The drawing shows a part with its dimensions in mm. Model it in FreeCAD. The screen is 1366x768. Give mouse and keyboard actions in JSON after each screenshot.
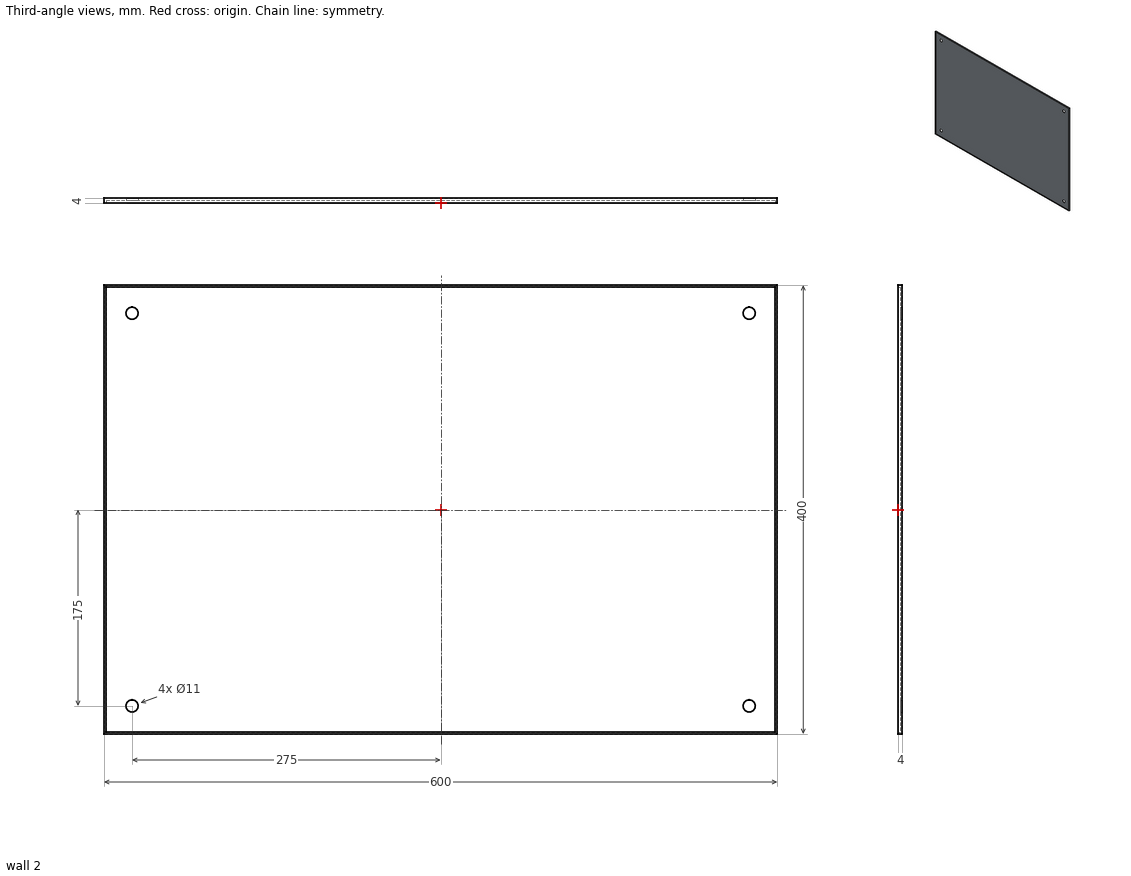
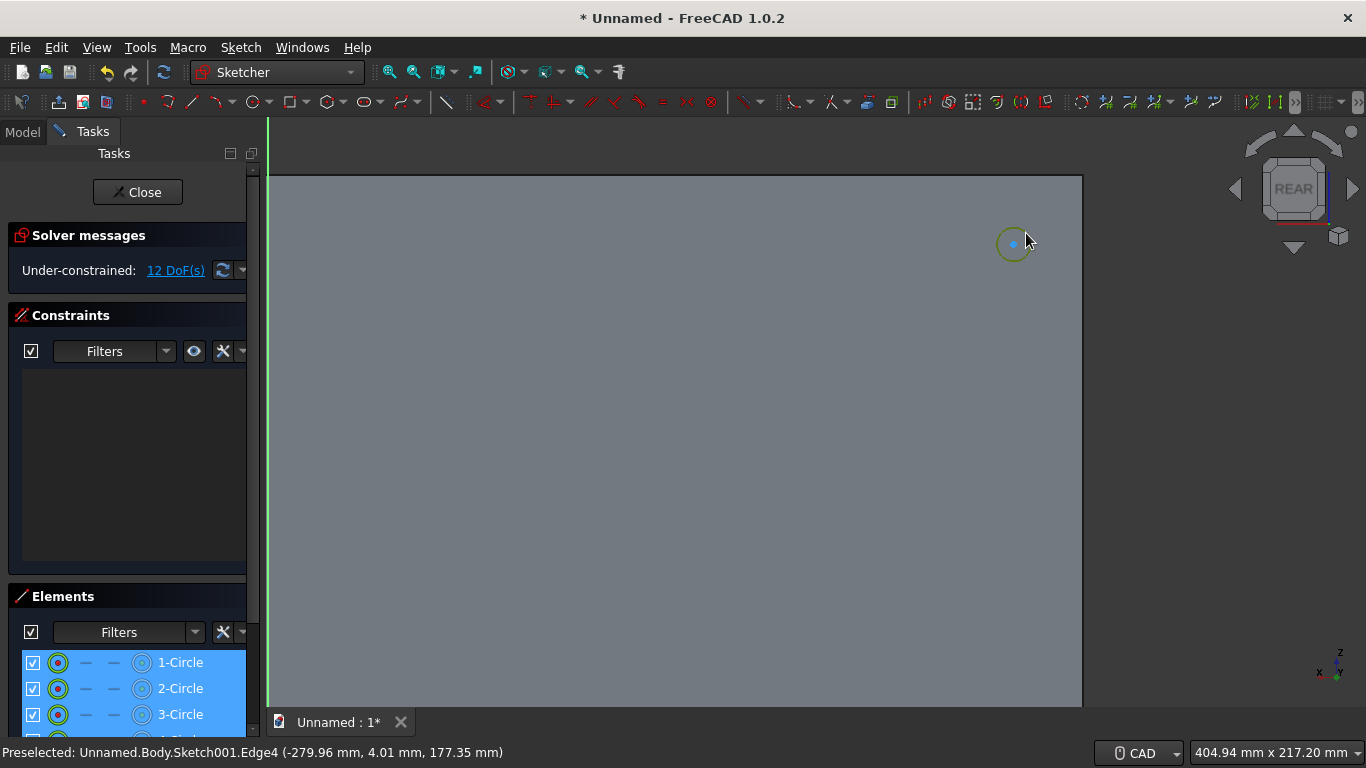
{"action": "key", "text": "e"}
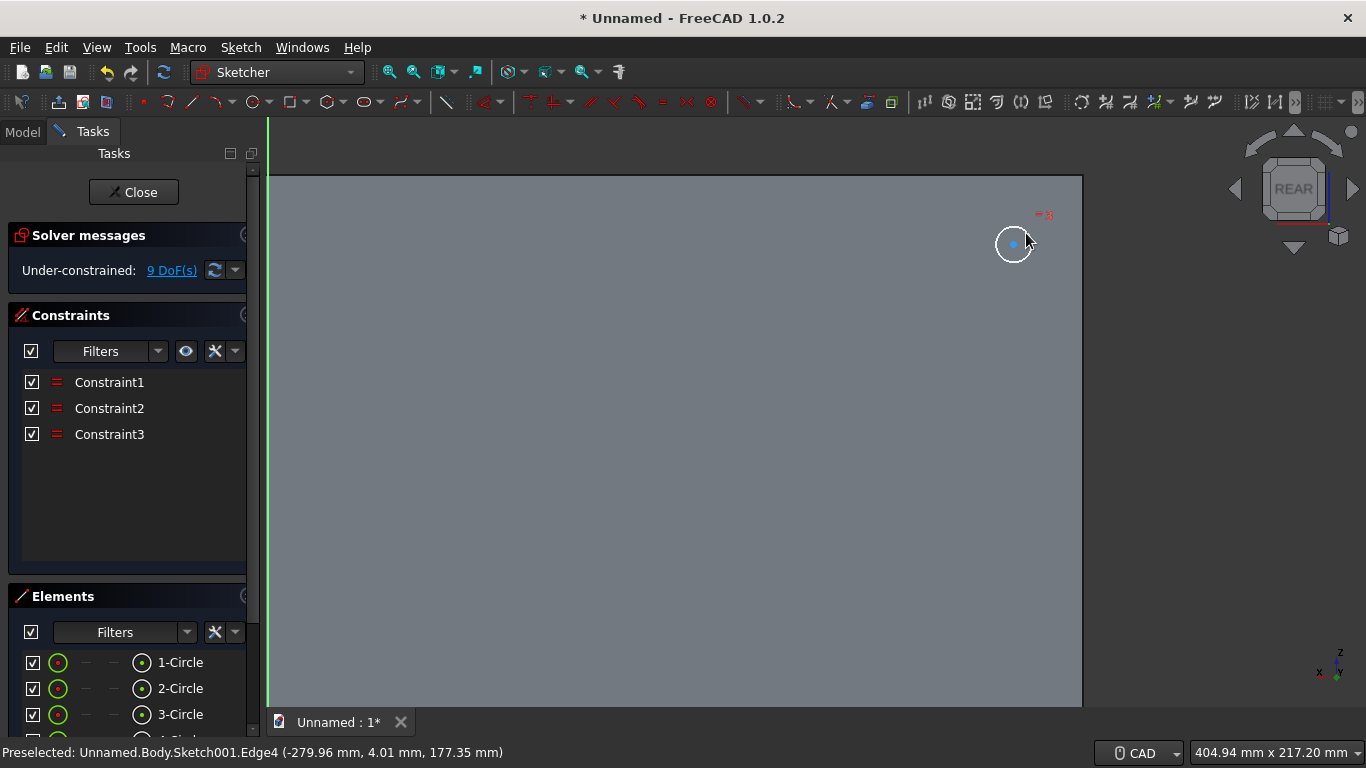
{"action": "scroll", "coordinate": [1026, 234], "scroll_direction": "down", "scroll_amount": 5}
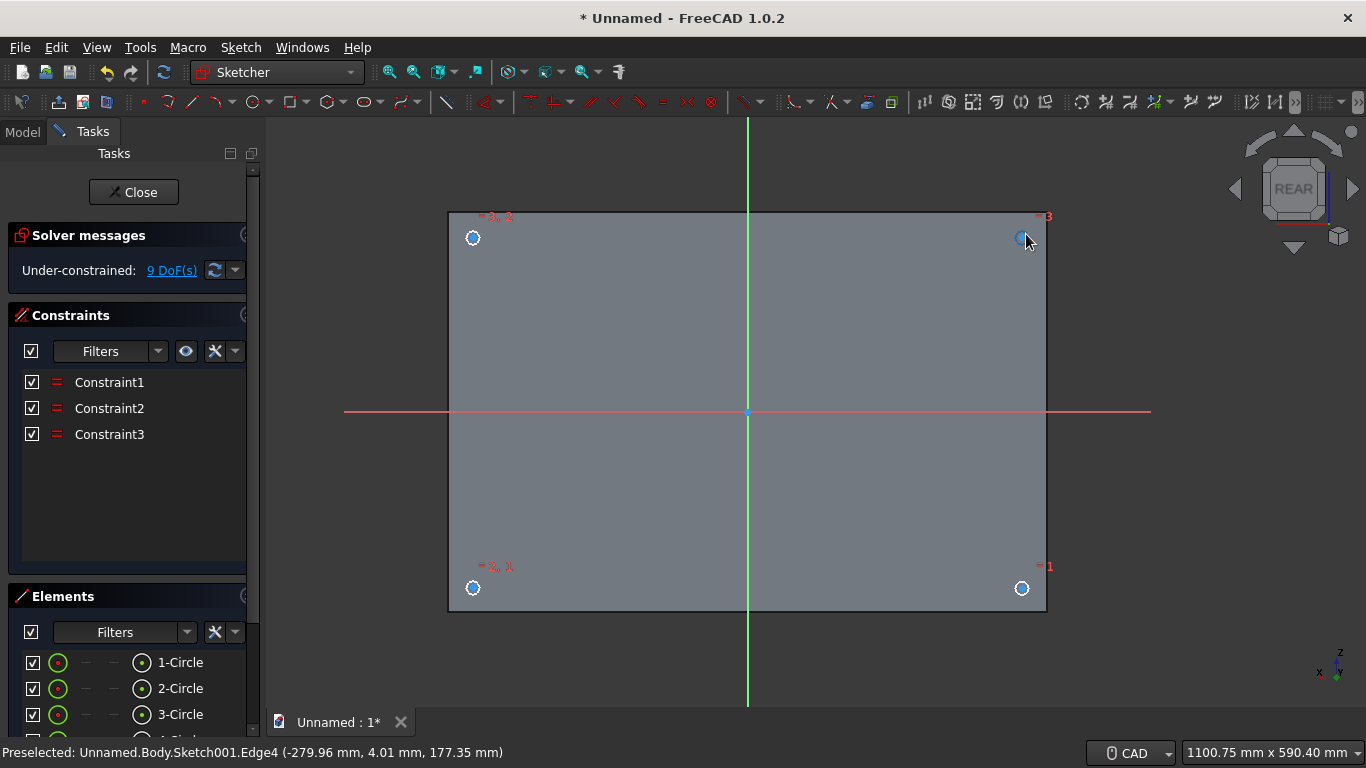
{"action": "left_click", "coordinate": [1022, 588]}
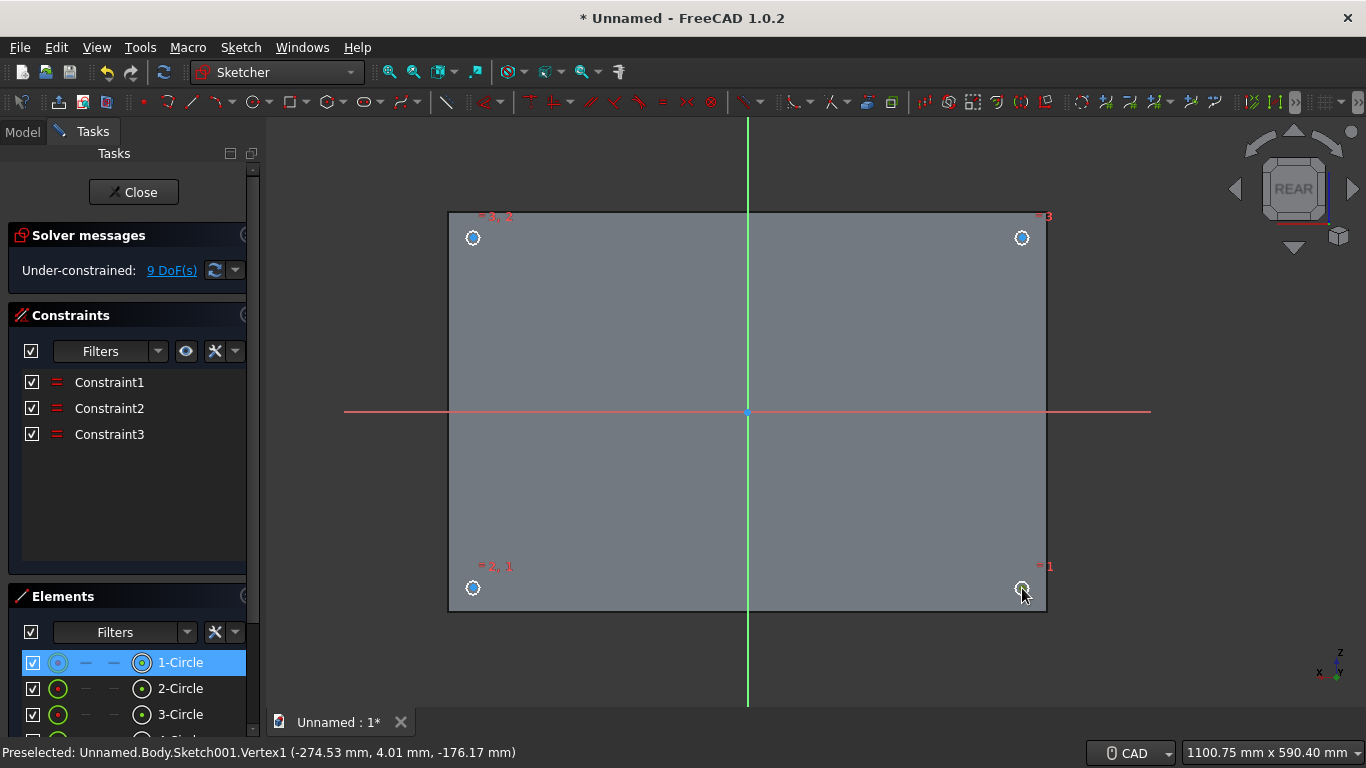
{"action": "left_click", "coordinate": [473, 588]}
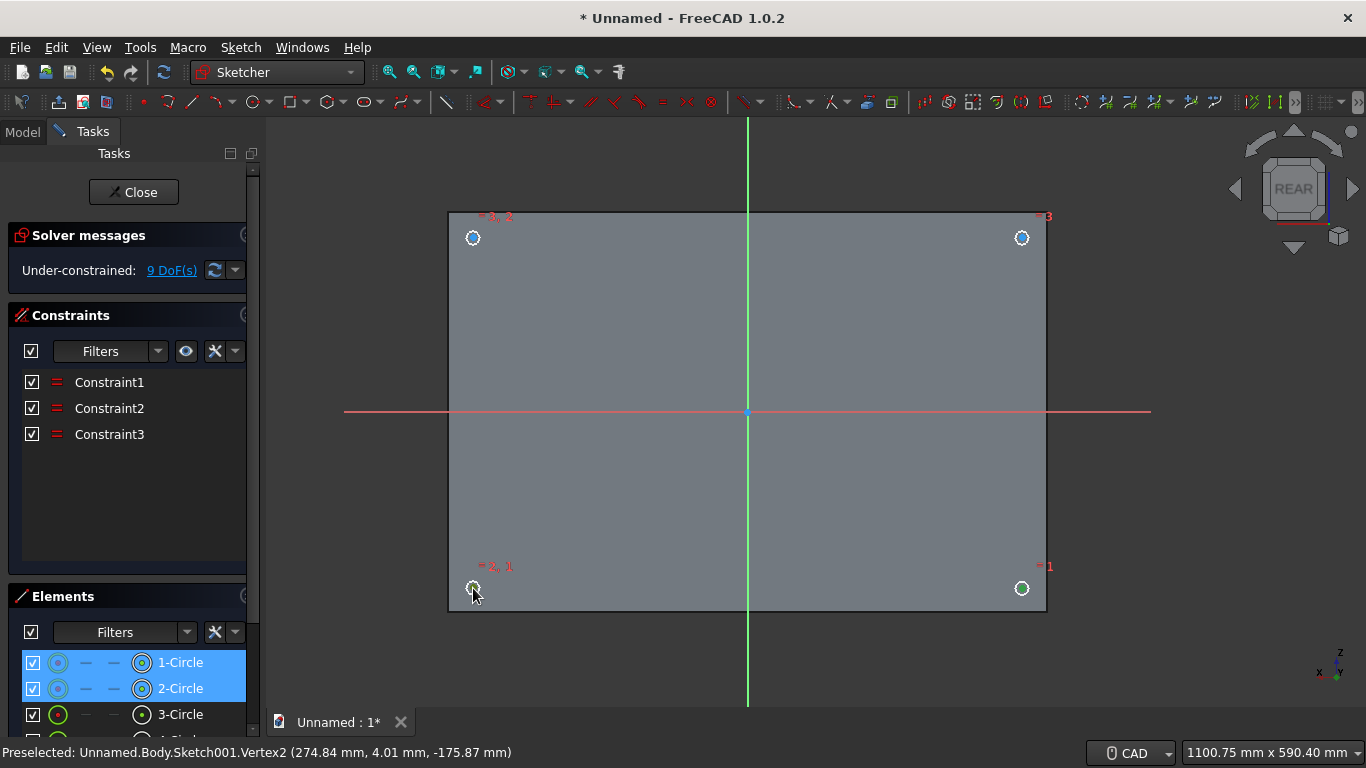
{"action": "left_click", "coordinate": [748, 641]}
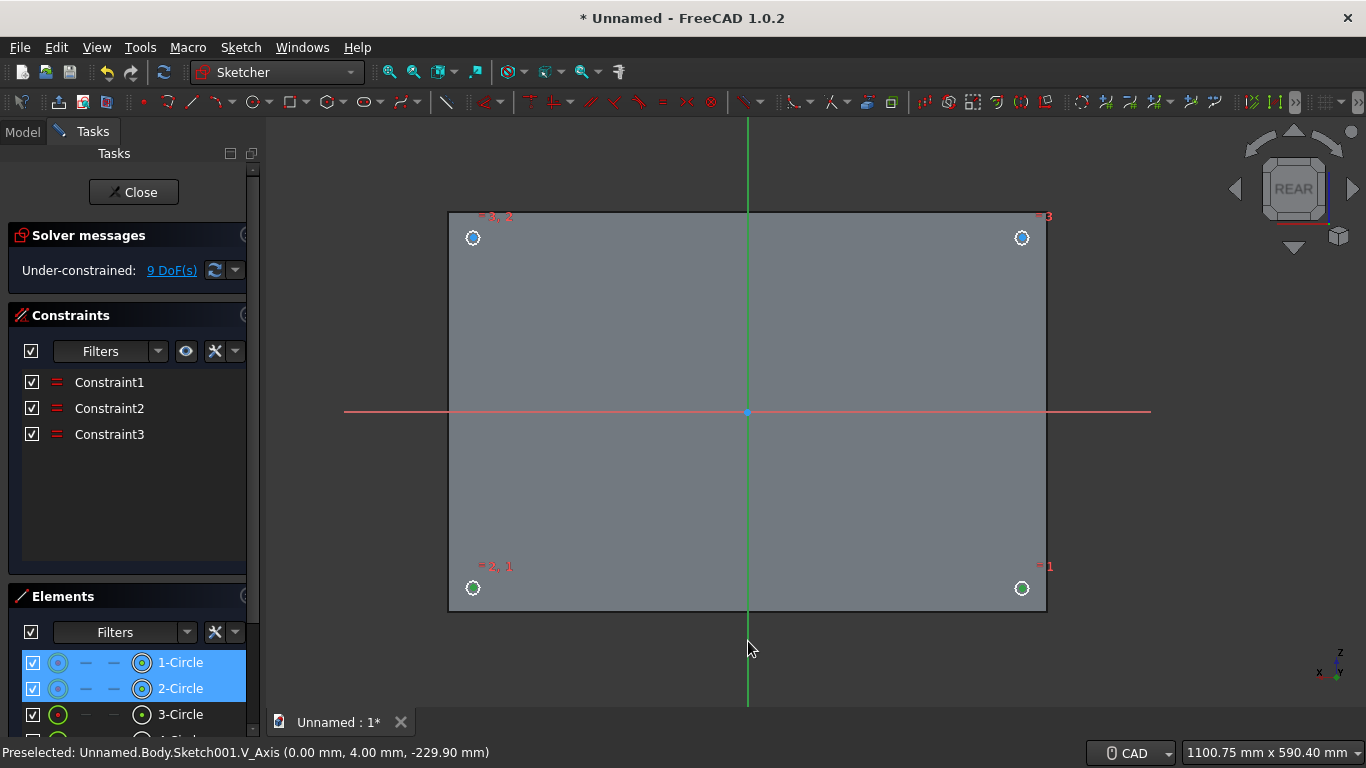
{"action": "key", "text": "s"}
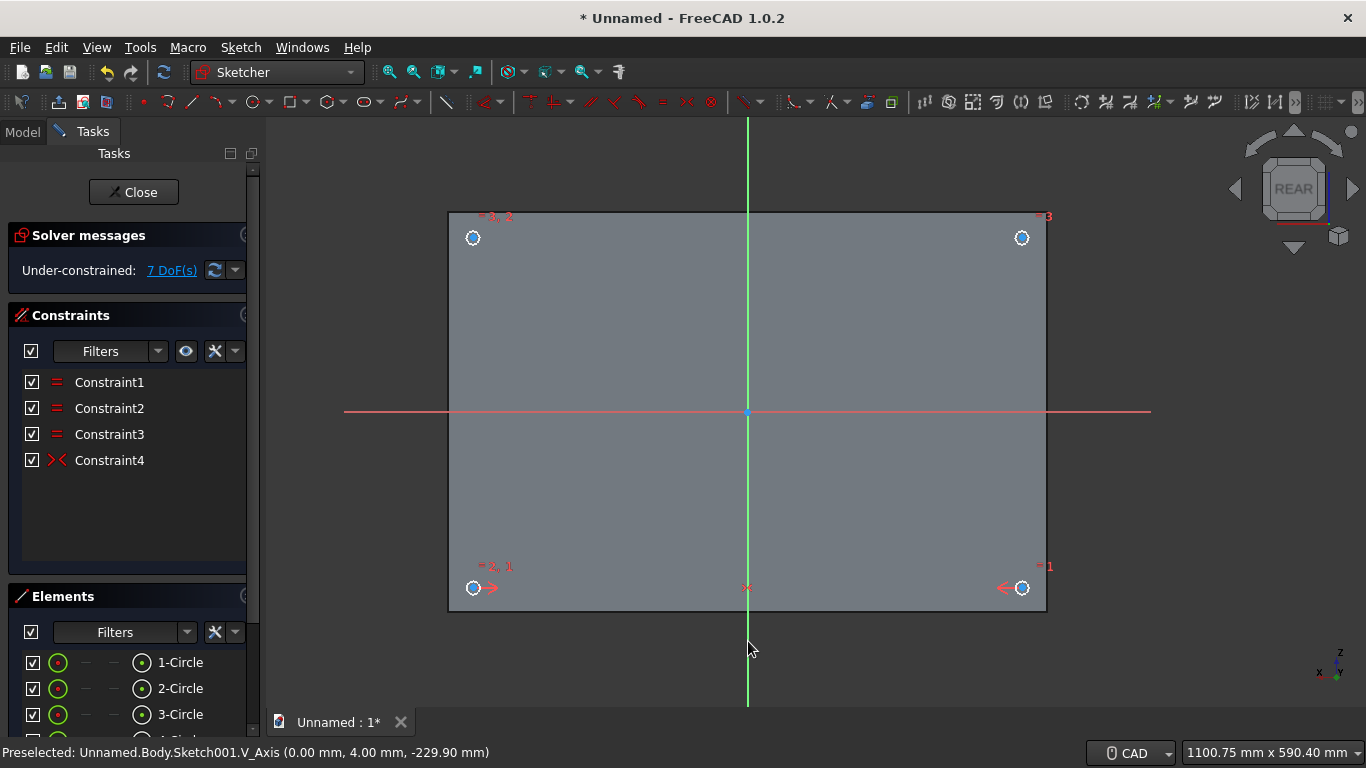
{"action": "left_click", "coordinate": [473, 588]}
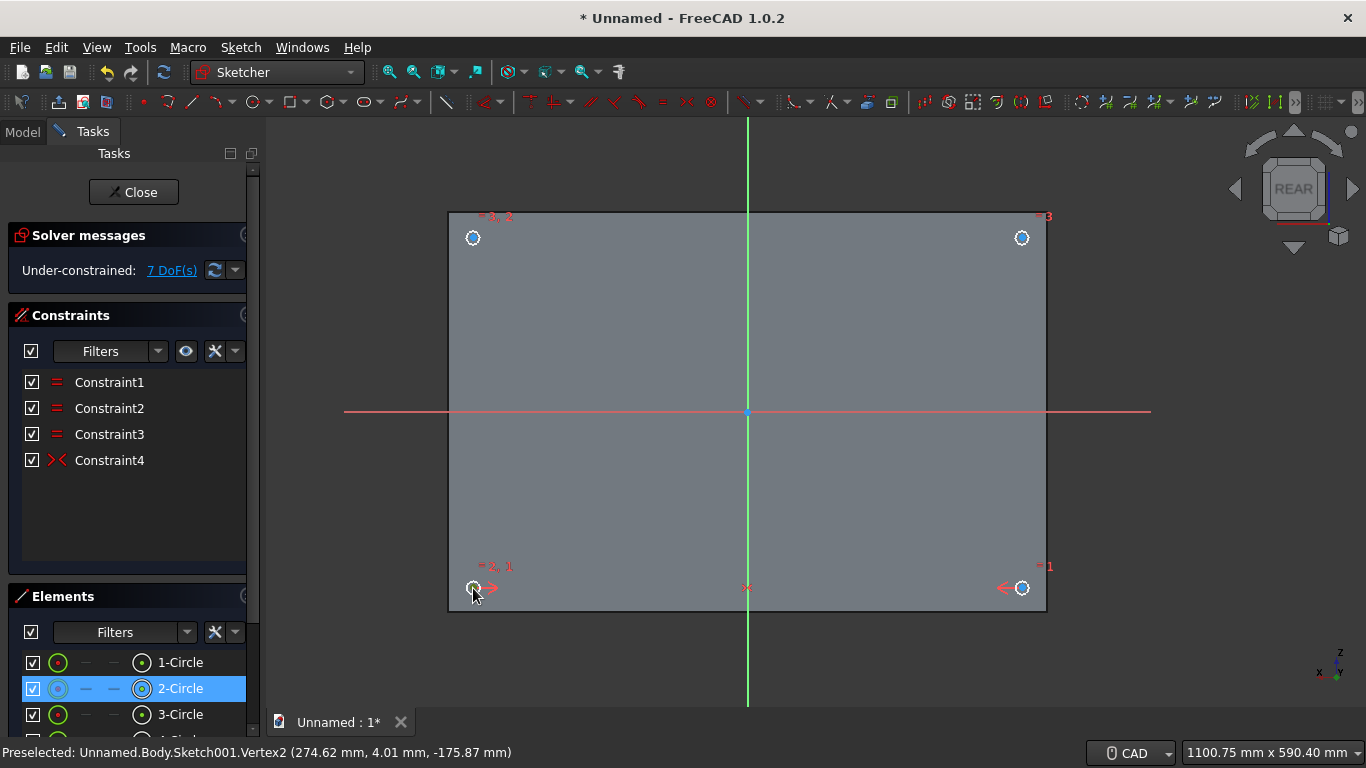
{"action": "left_click", "coordinate": [473, 238]}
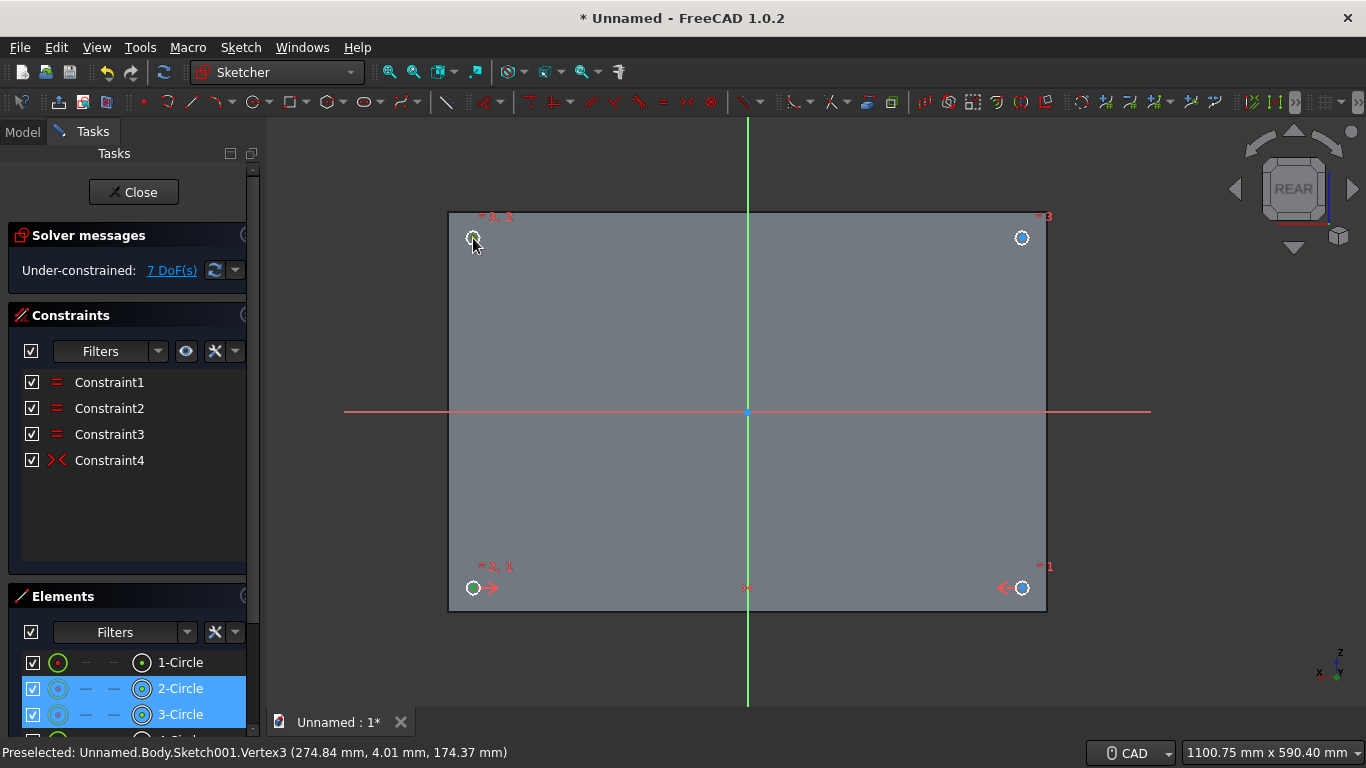
{"action": "left_click", "coordinate": [359, 412]}